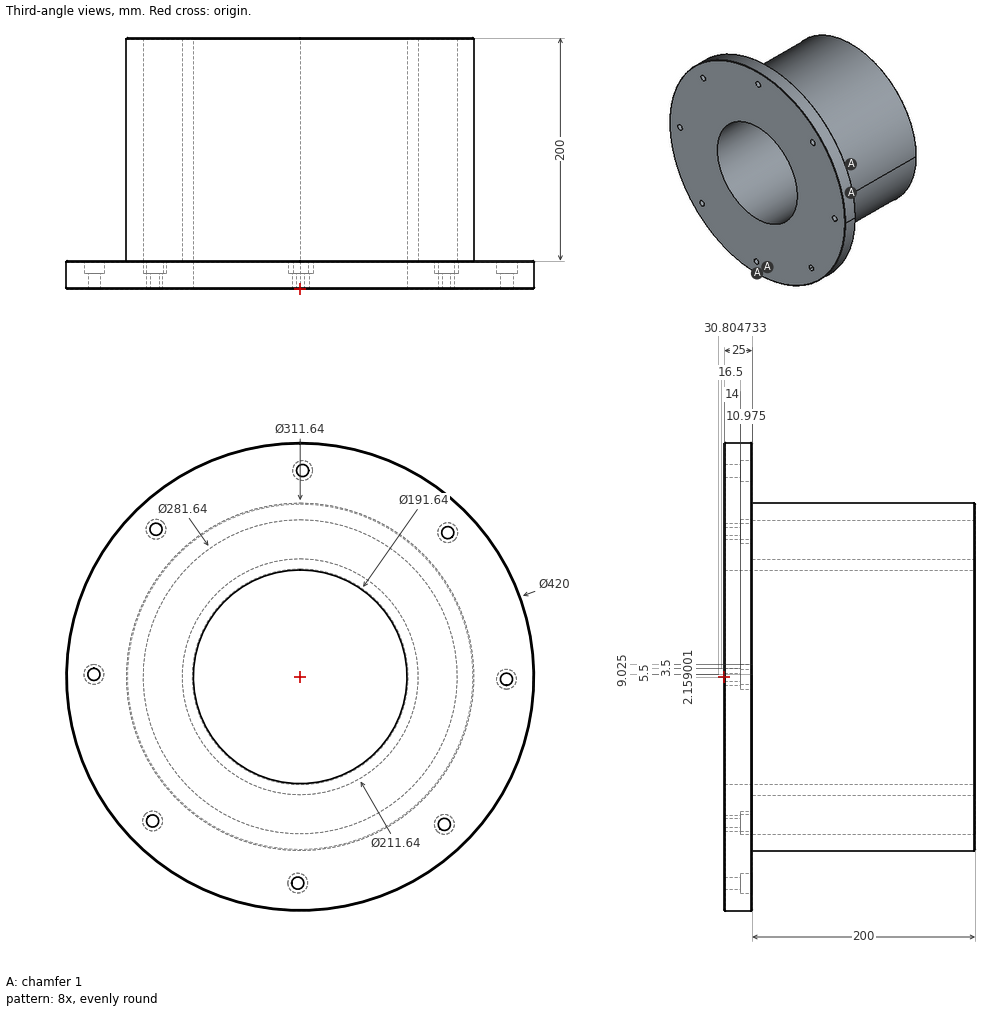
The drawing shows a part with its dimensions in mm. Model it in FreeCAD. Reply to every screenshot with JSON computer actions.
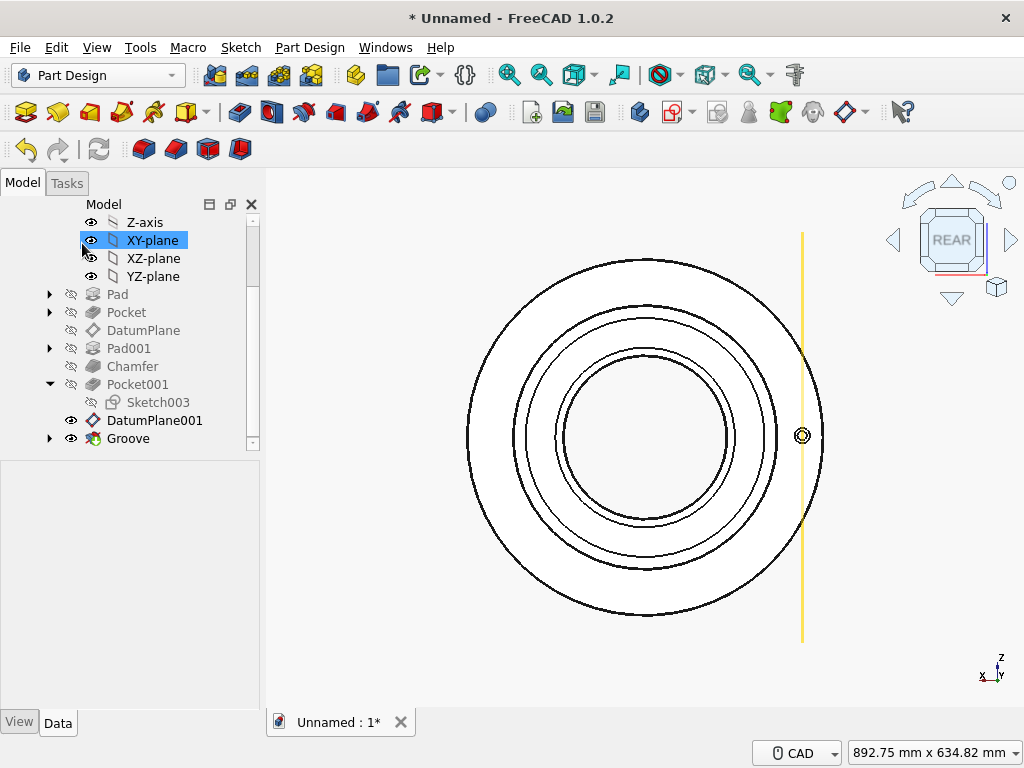
{"action": "left_click", "coordinate": [116, 420]}
{"action": "key", "text": "space"}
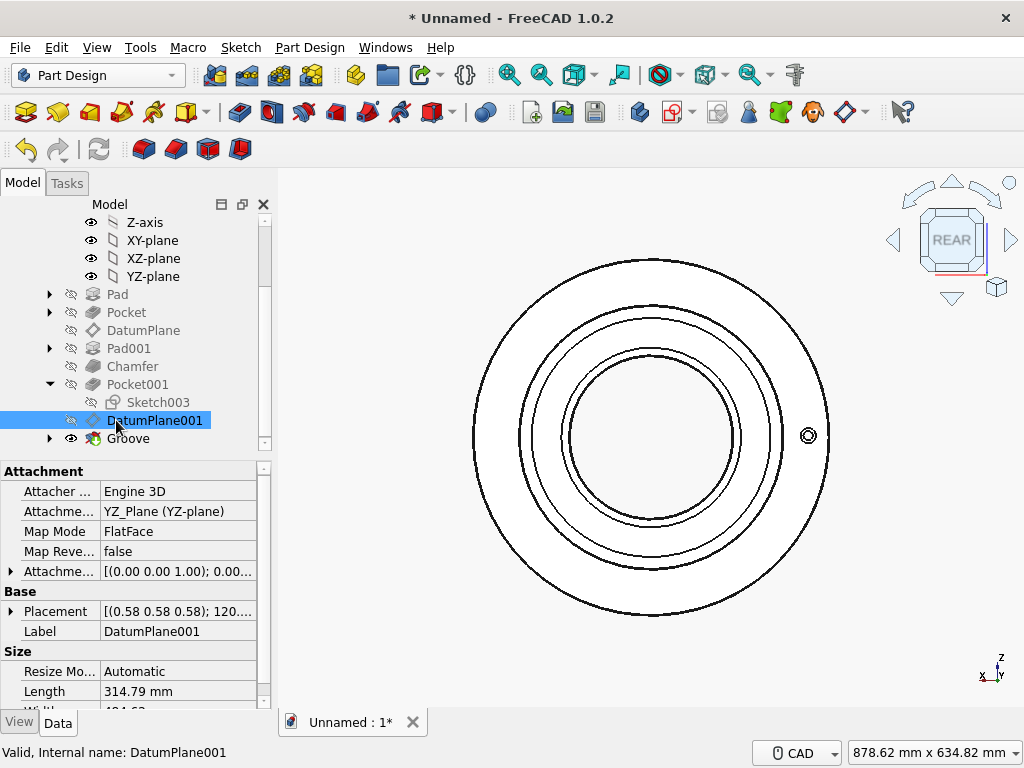
{"action": "left_click", "coordinate": [116, 438]}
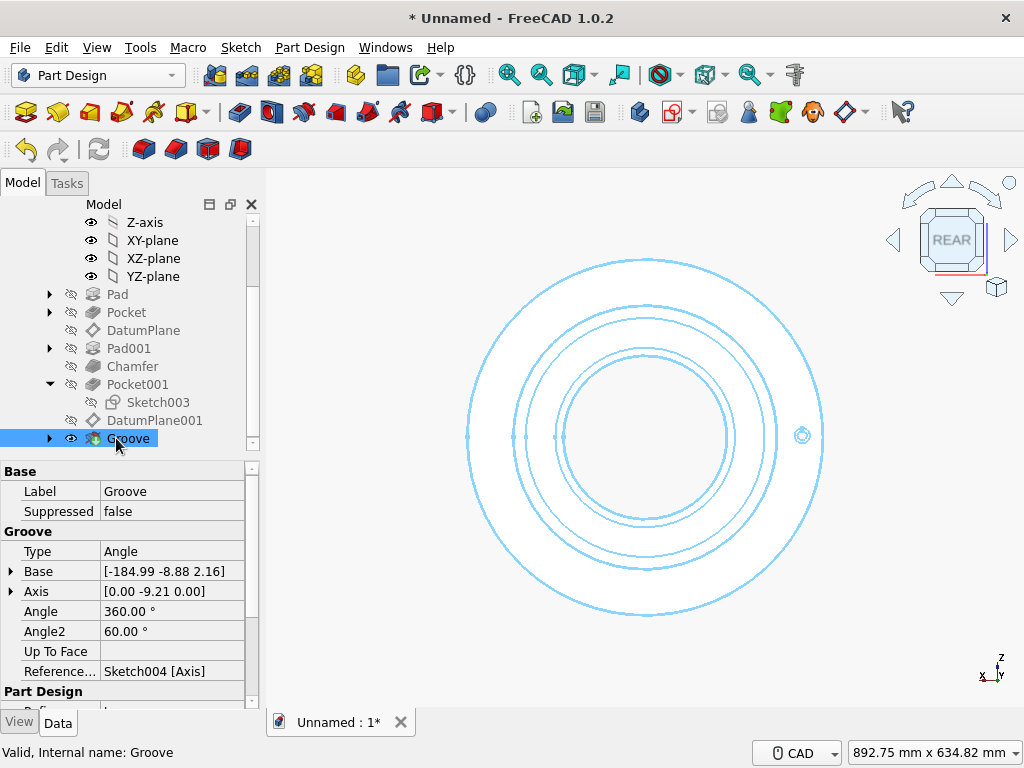
{"action": "left_click", "coordinate": [280, 76]}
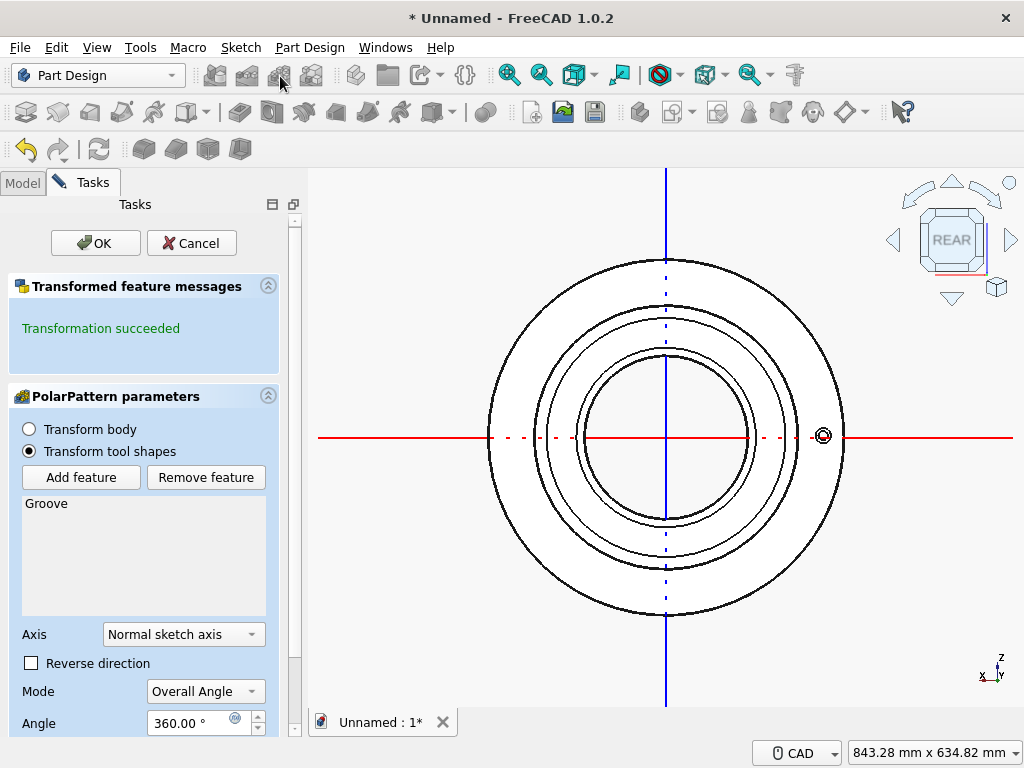
{"action": "left_click", "coordinate": [184, 634]}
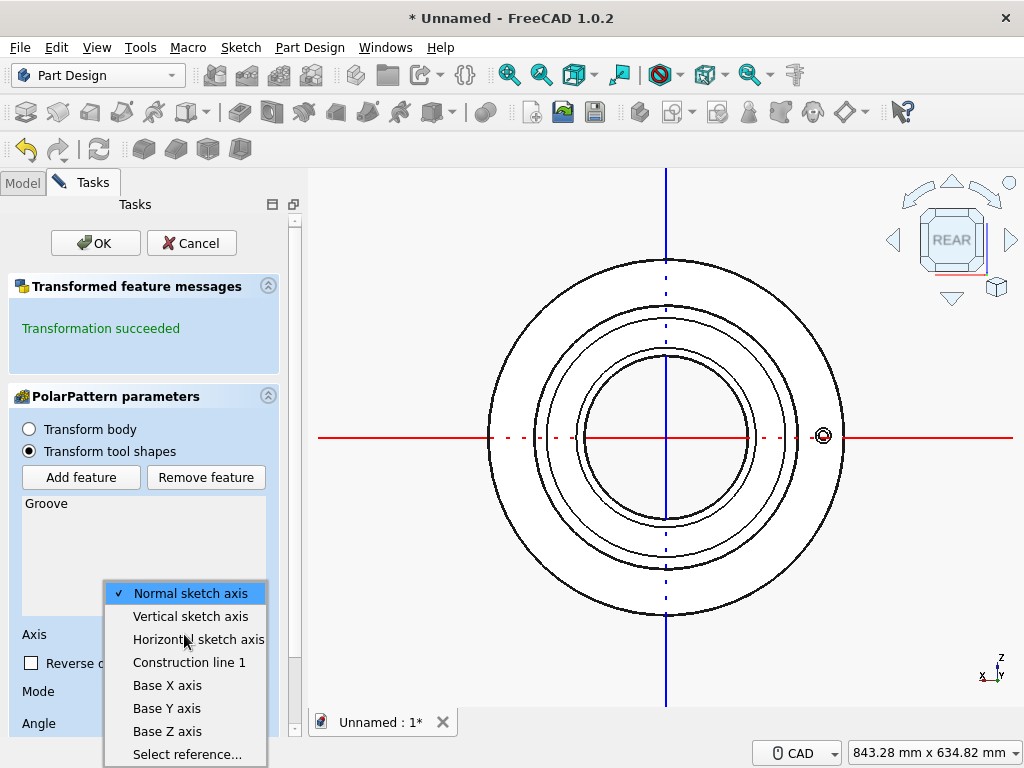
{"action": "left_click", "coordinate": [184, 708]}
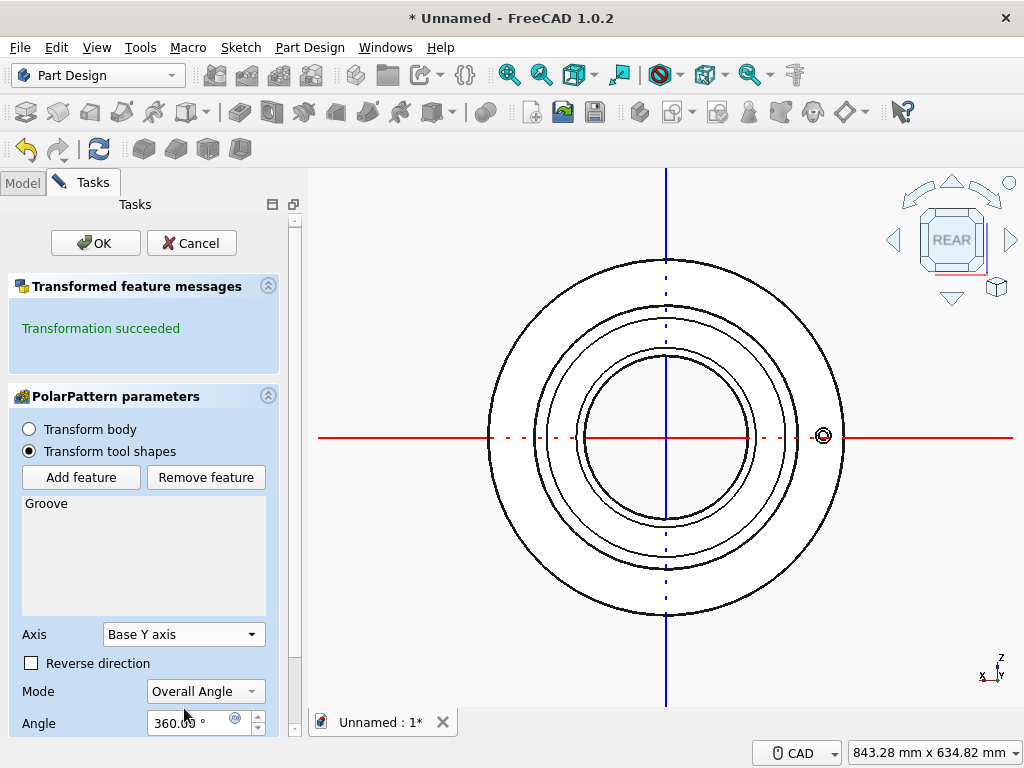
{"action": "scroll", "coordinate": [295, 475], "scroll_direction": "down", "scroll_amount": 2}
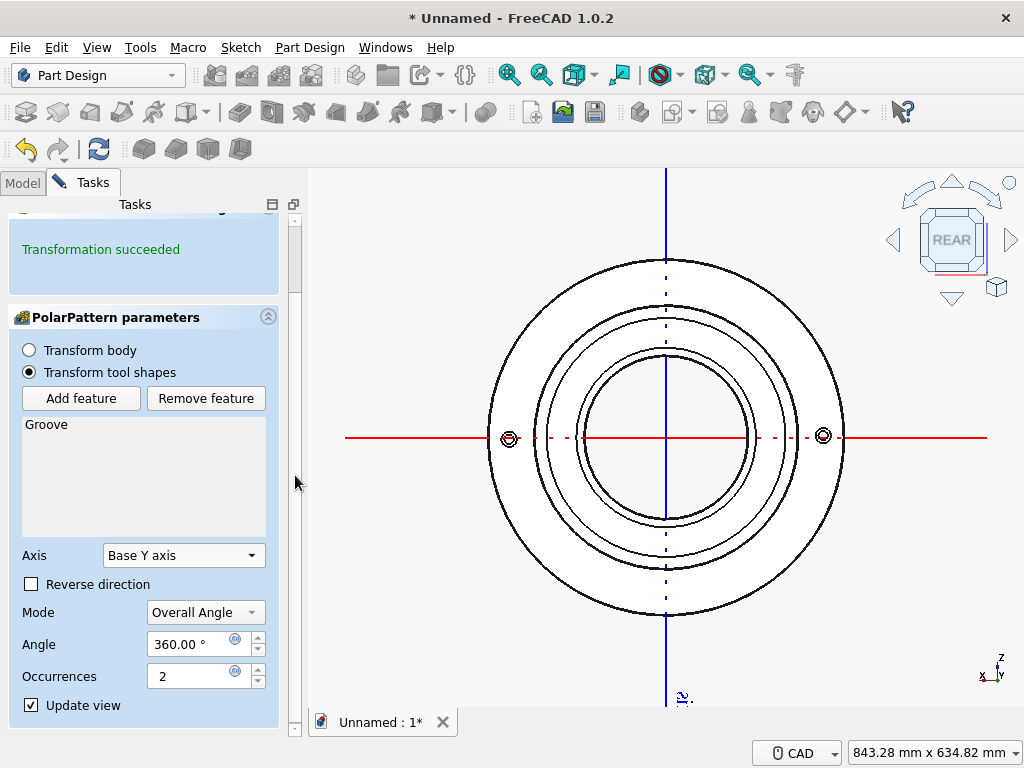
{"action": "triple_click", "coordinate": [198, 676]}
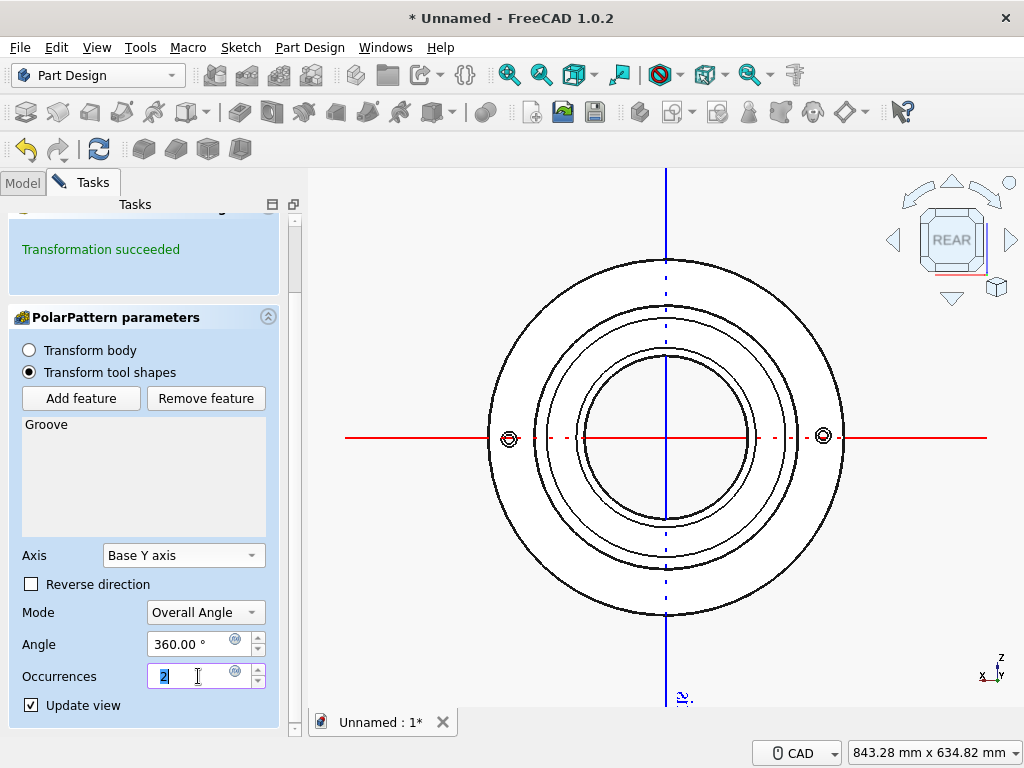
{"action": "type", "text": "8"}
{"action": "key", "text": "Tab"}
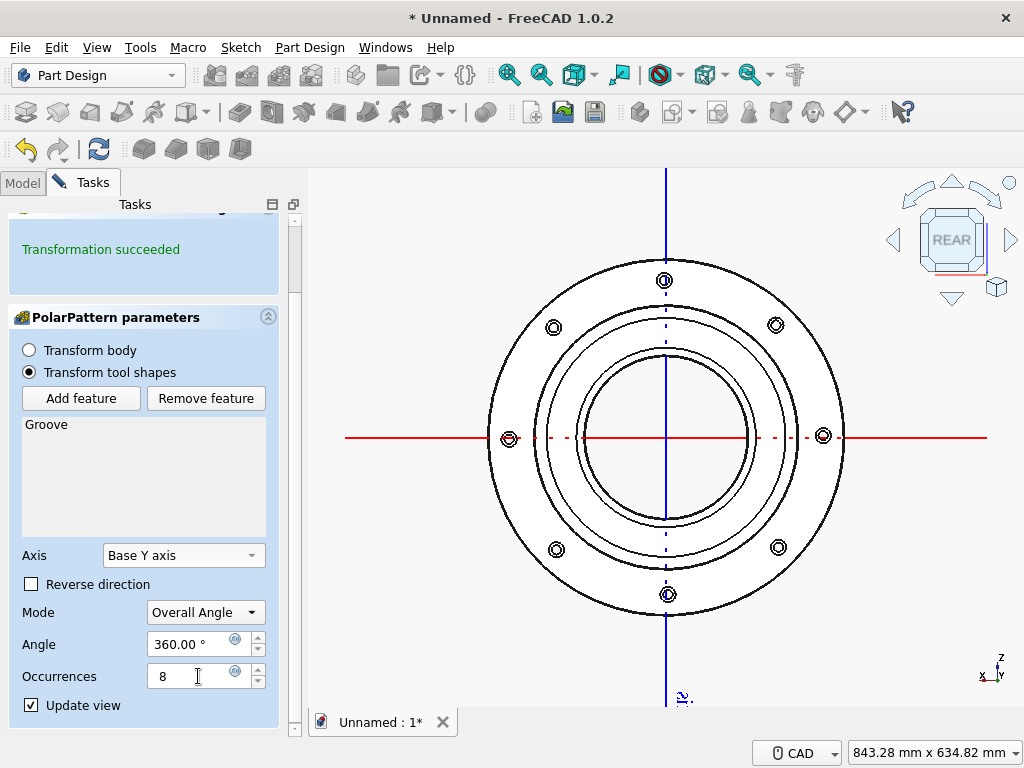
{"action": "scroll", "coordinate": [295, 475], "scroll_direction": "up", "scroll_amount": 3}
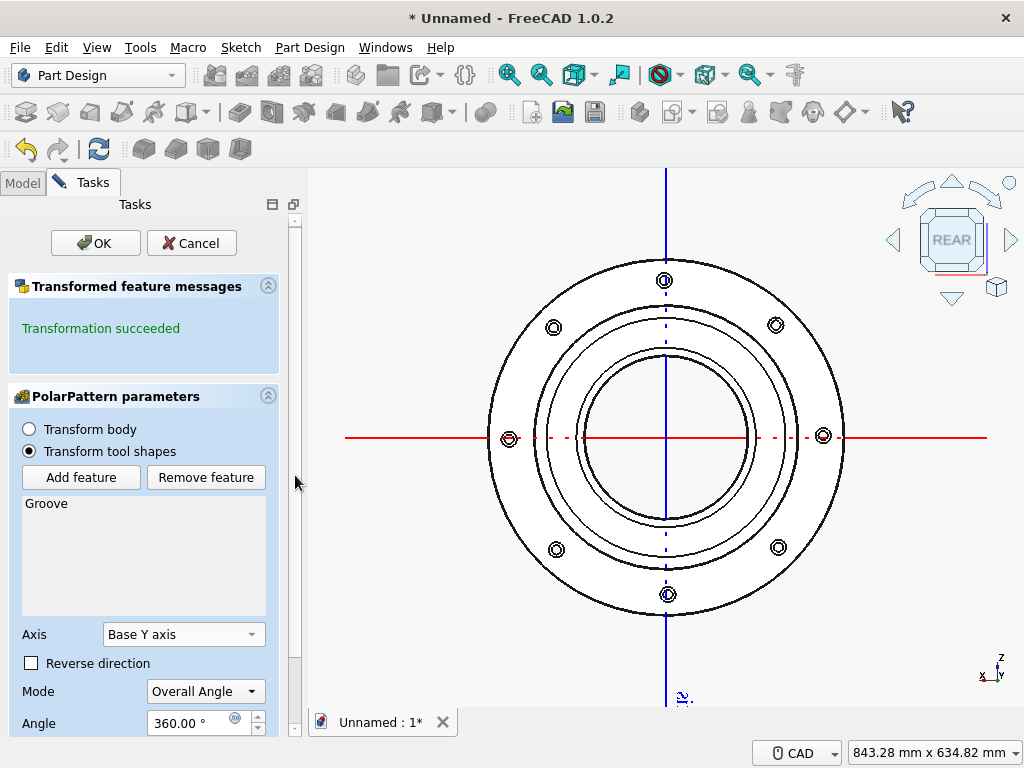
{"action": "left_click", "coordinate": [96, 243]}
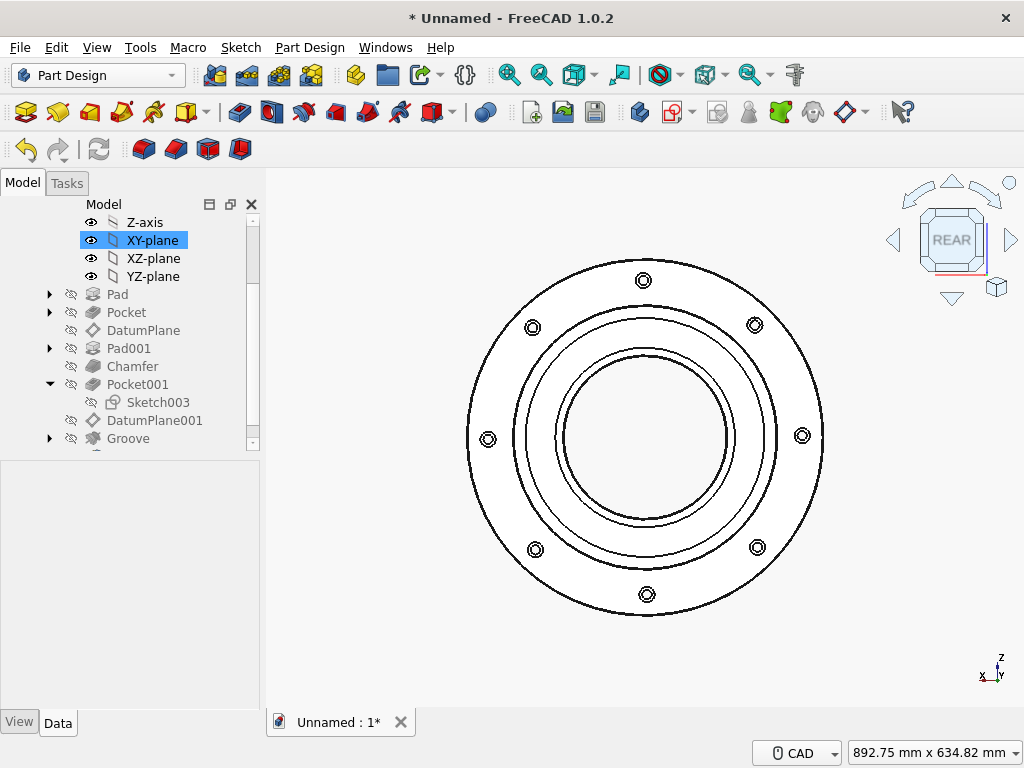
{"action": "key", "text": "0"}